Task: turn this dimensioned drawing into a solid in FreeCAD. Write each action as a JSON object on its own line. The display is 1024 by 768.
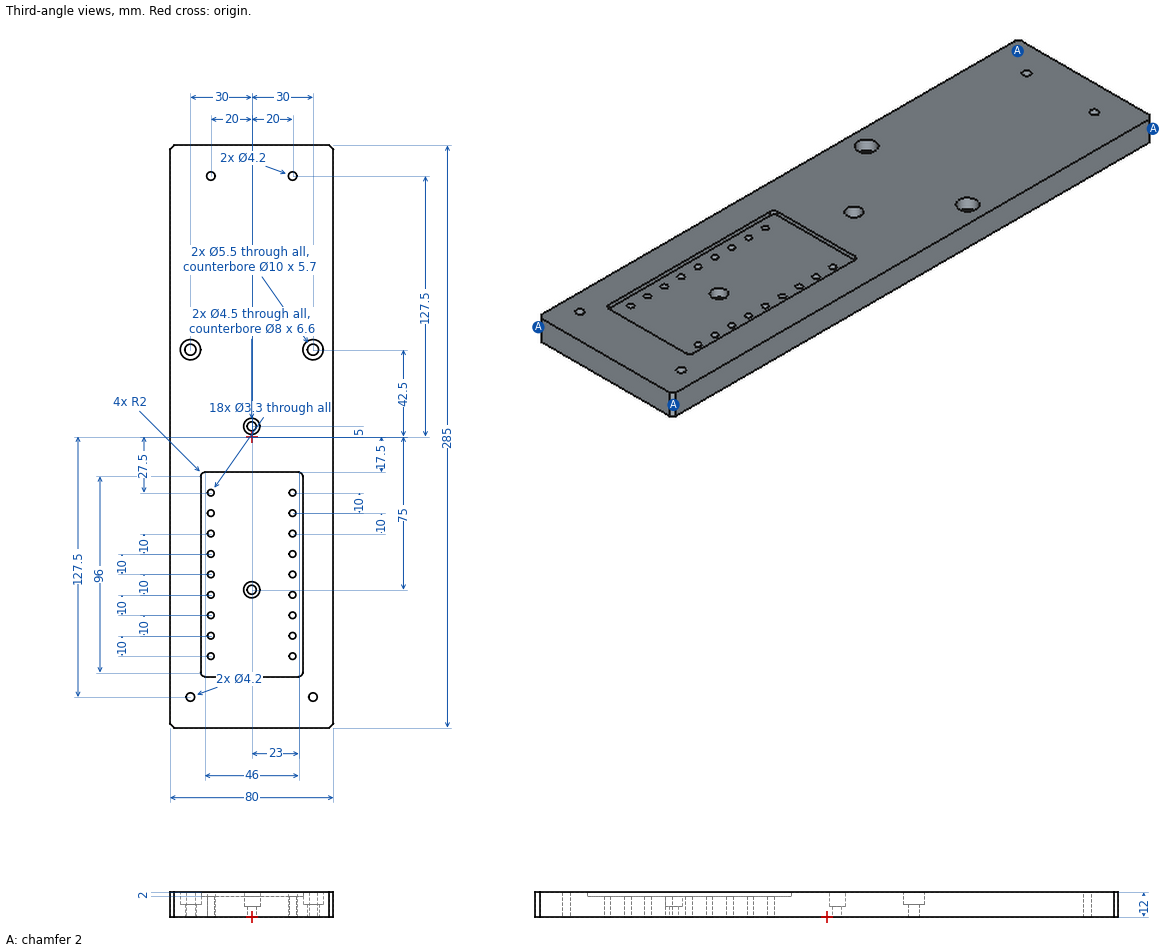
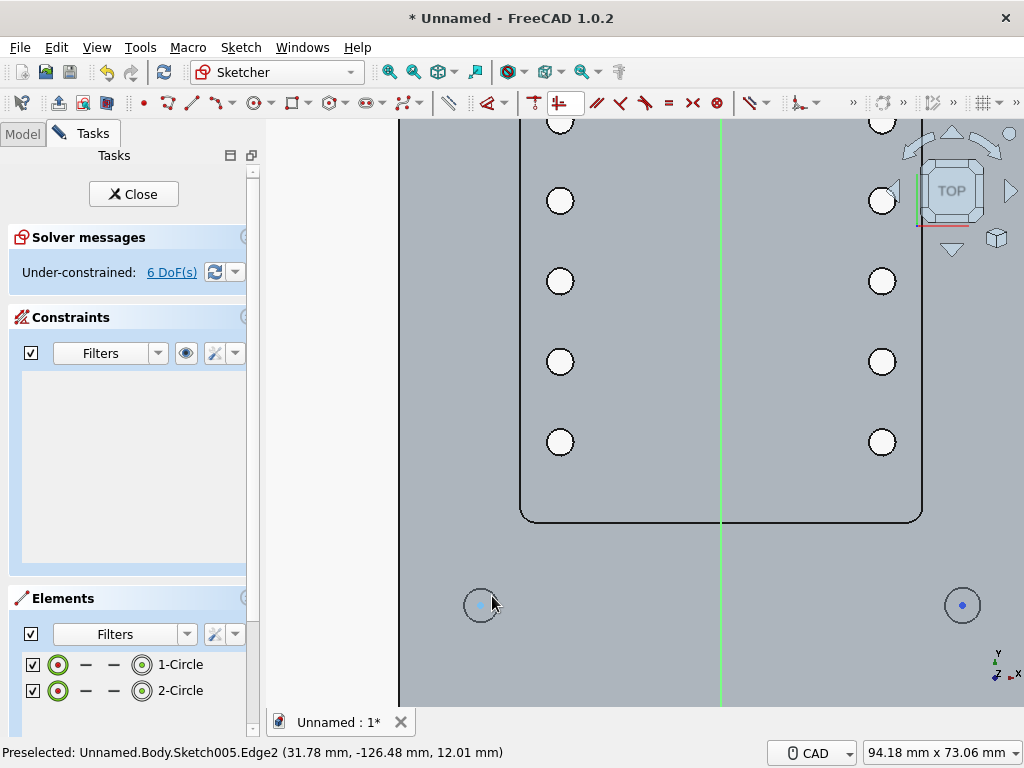
{"action": "left_click", "coordinate": [493, 594]}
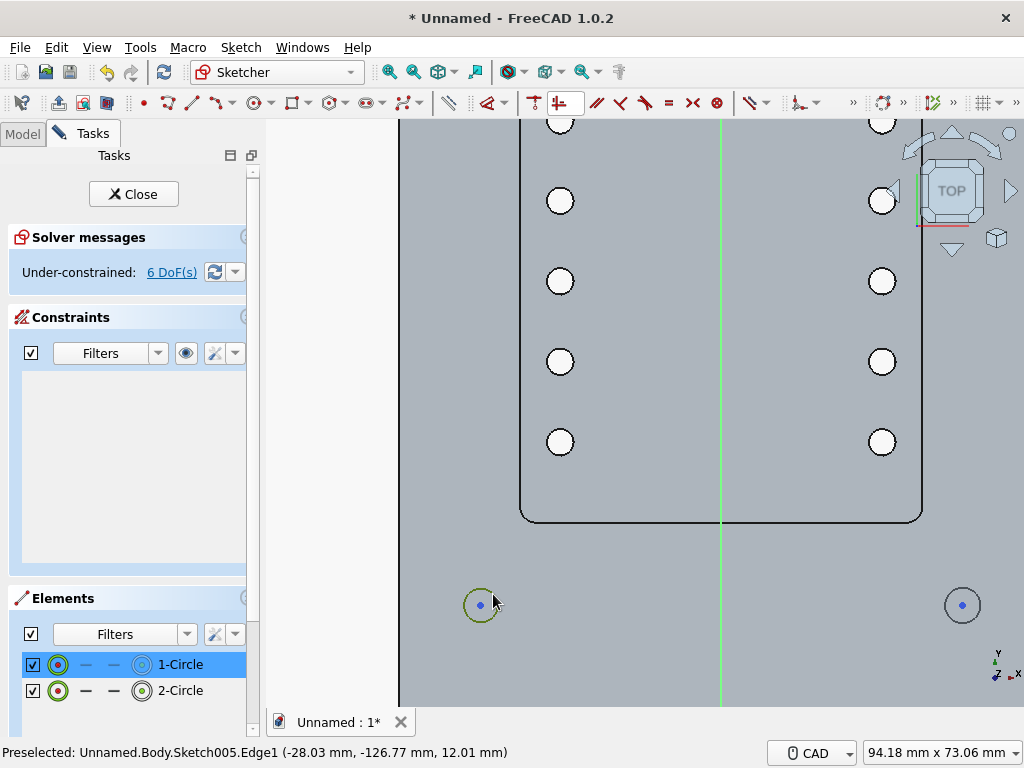
{"action": "scroll", "coordinate": [492, 596], "scroll_direction": "down", "scroll_amount": 5}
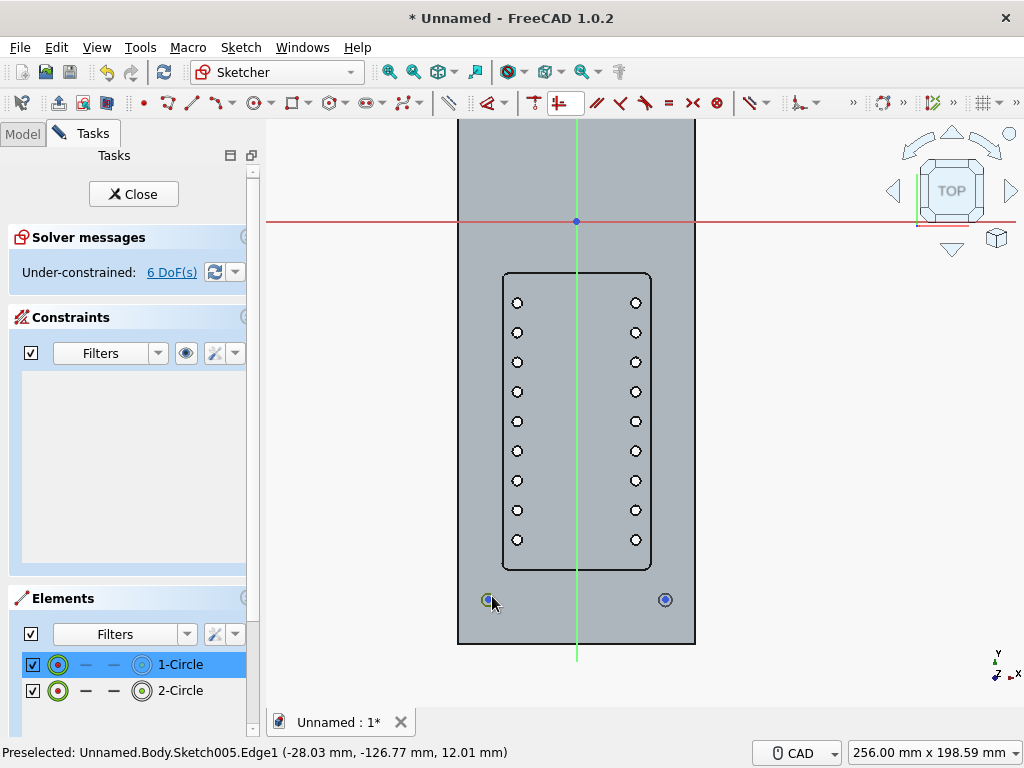
{"action": "scroll", "coordinate": [670, 595], "scroll_direction": "up", "scroll_amount": 4}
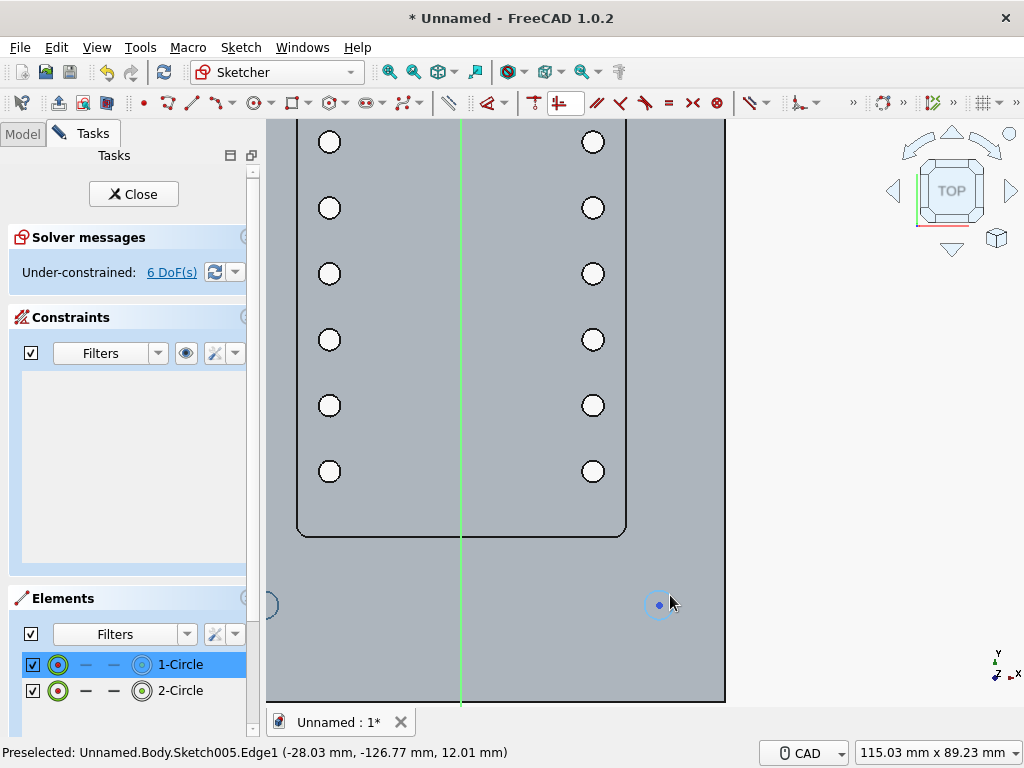
{"action": "left_click", "coordinate": [669, 595]}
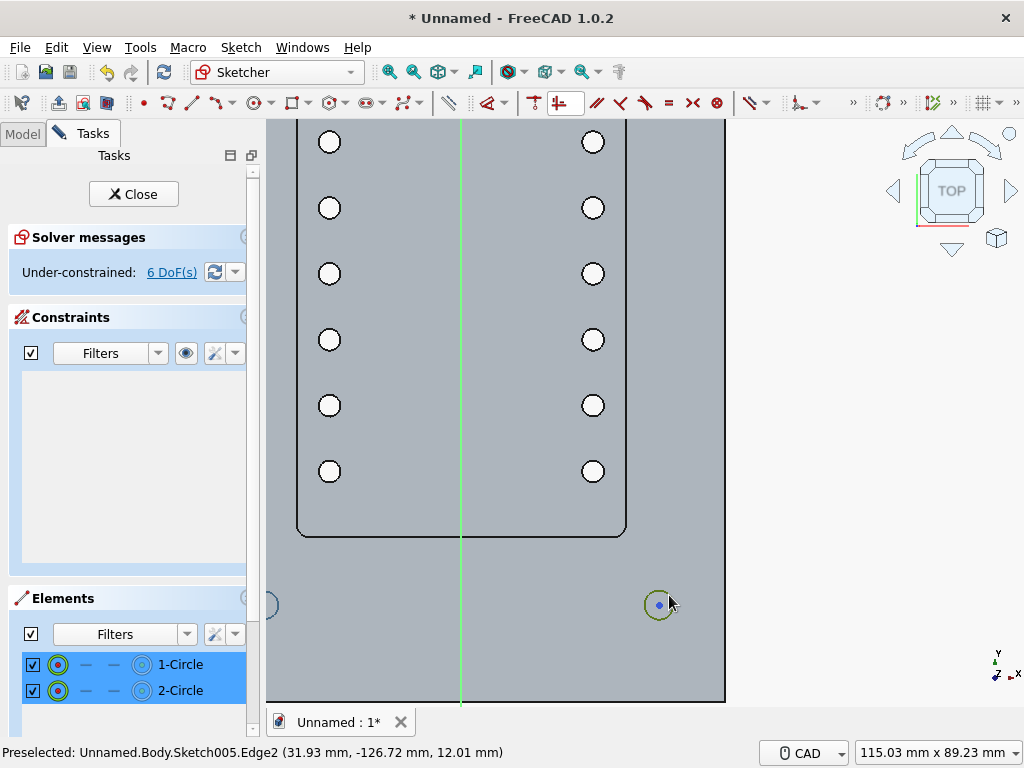
{"action": "key", "text": "e"}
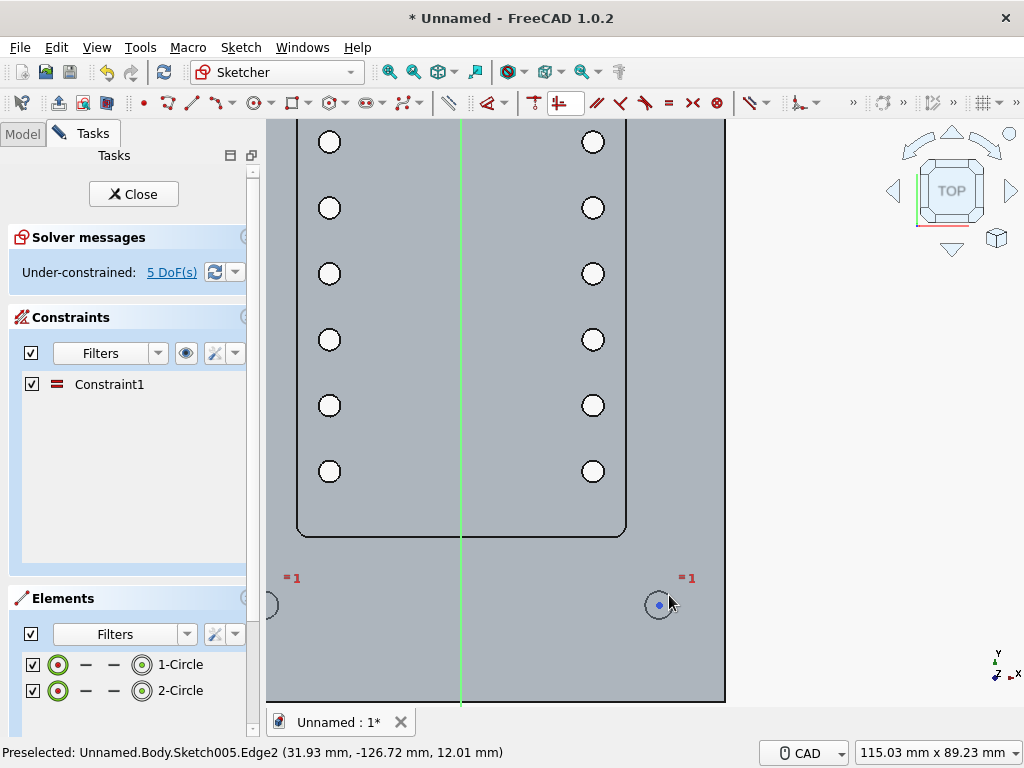
{"action": "scroll", "coordinate": [670, 595], "scroll_direction": "down", "scroll_amount": 4}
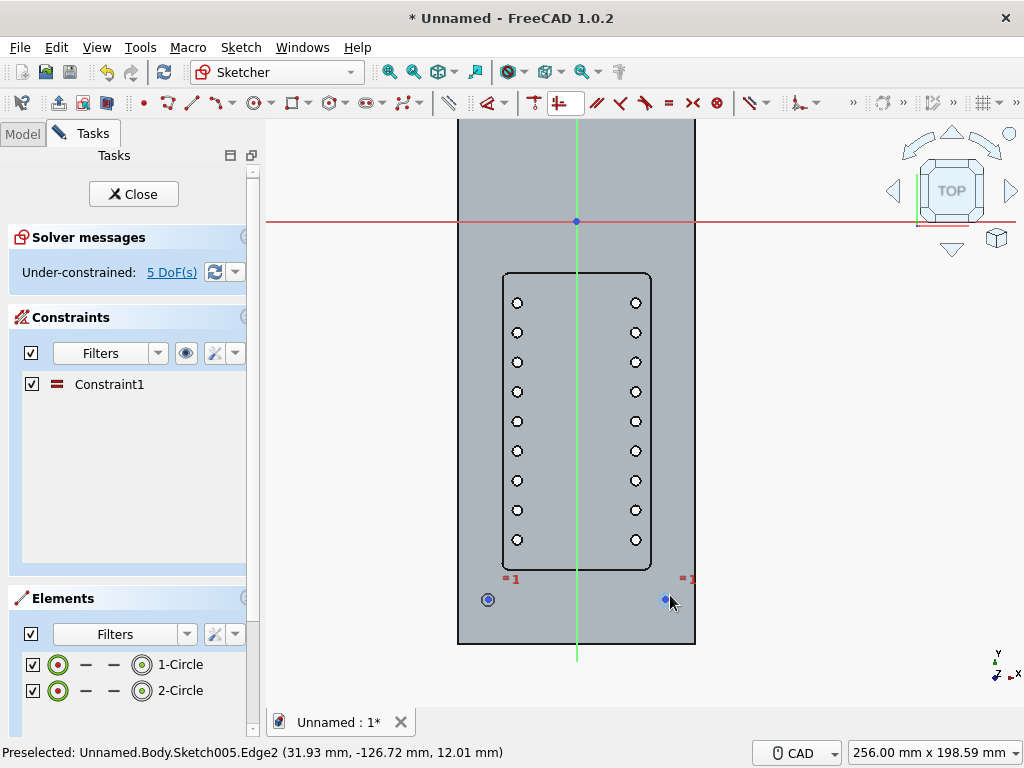
{"action": "left_click", "coordinate": [488, 600]}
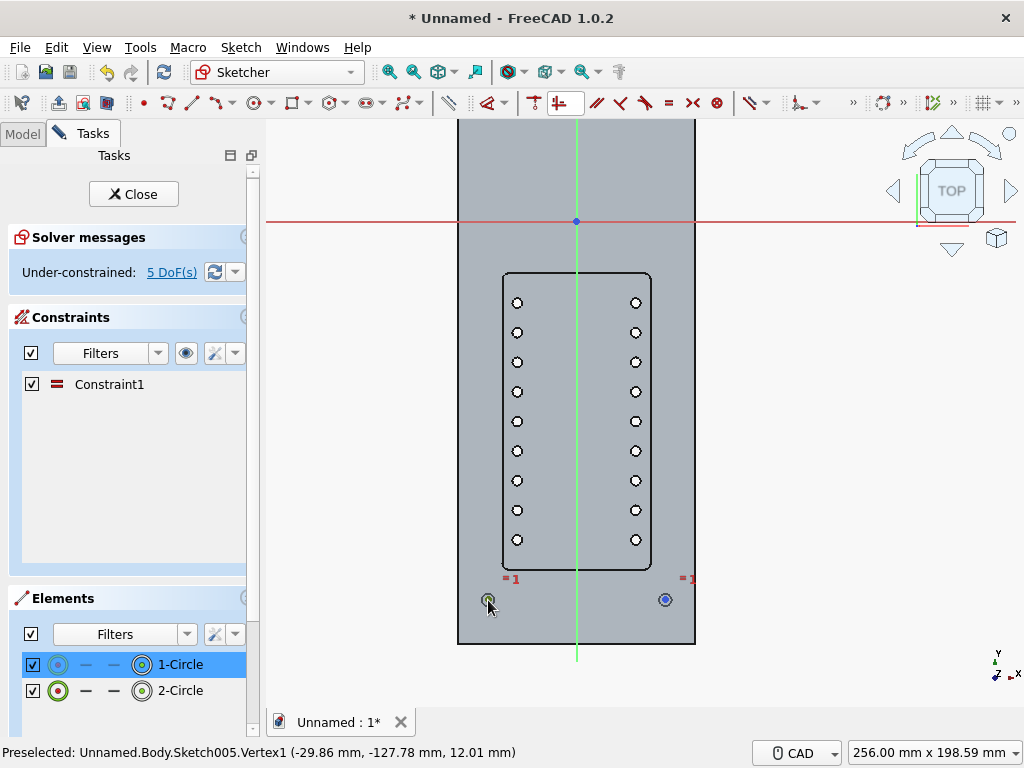
{"action": "left_click", "coordinate": [665, 600]}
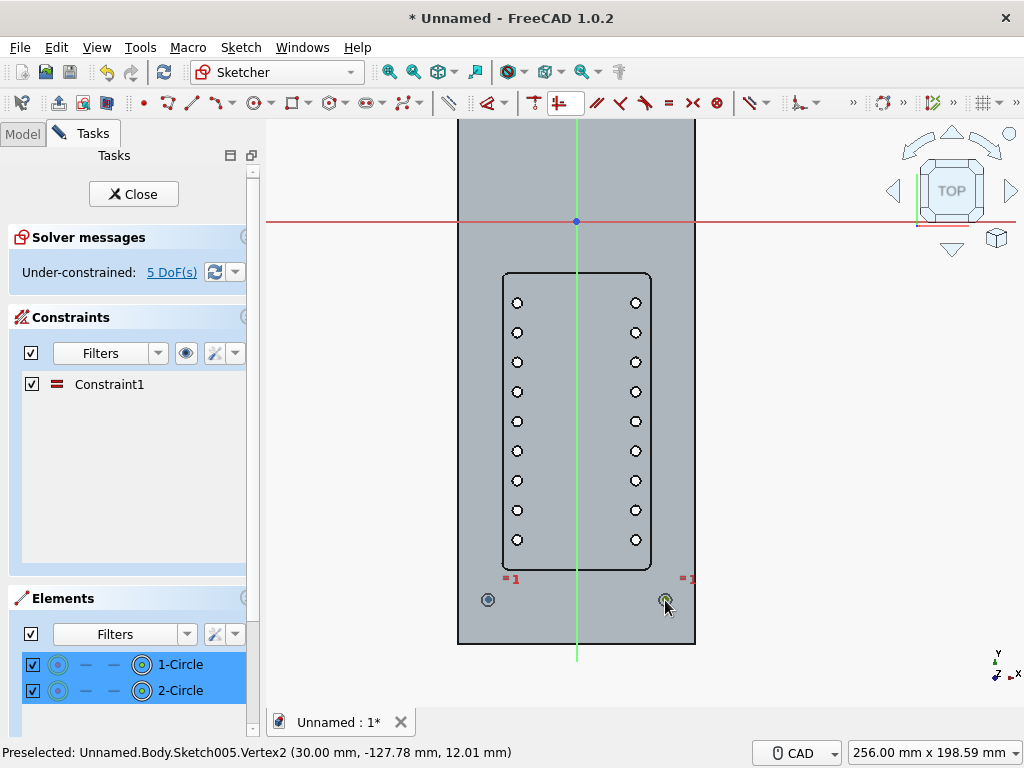
{"action": "key", "text": "h"}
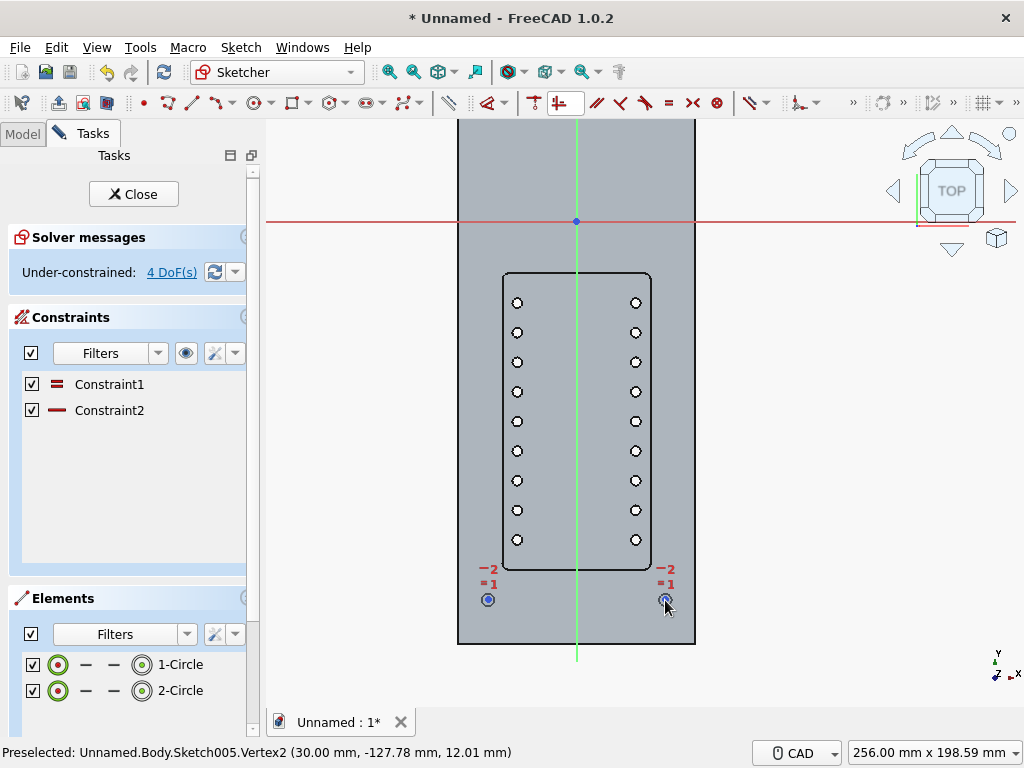
{"action": "key", "text": "d"}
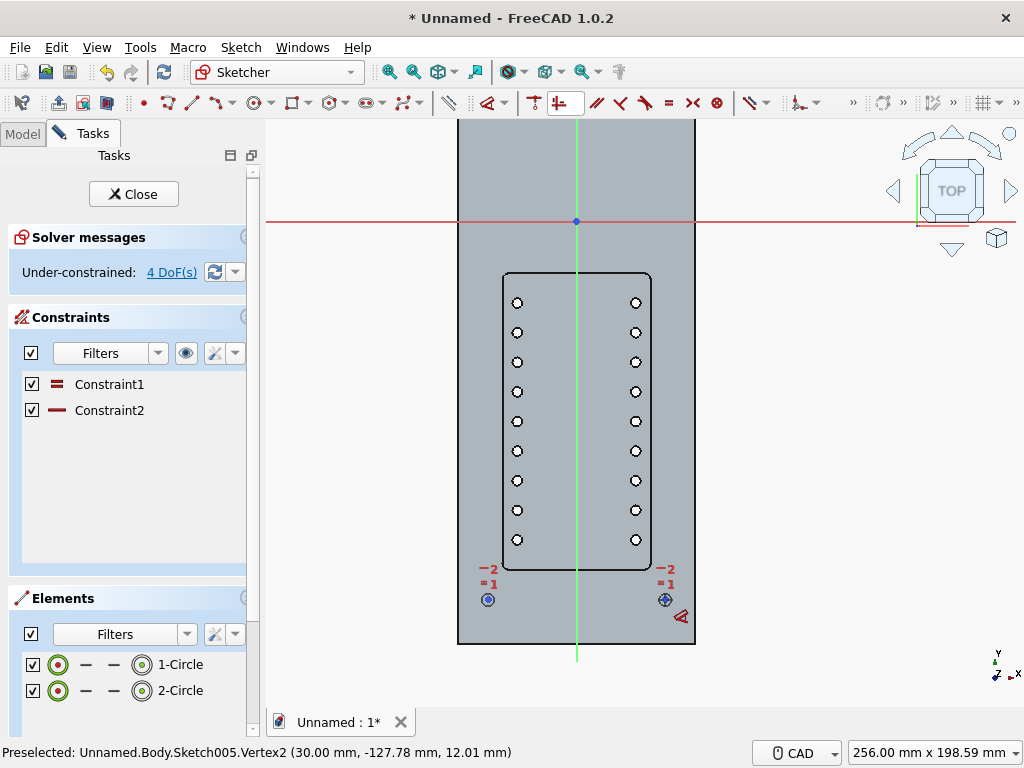
{"action": "scroll", "coordinate": [488, 606], "scroll_direction": "up", "scroll_amount": 6}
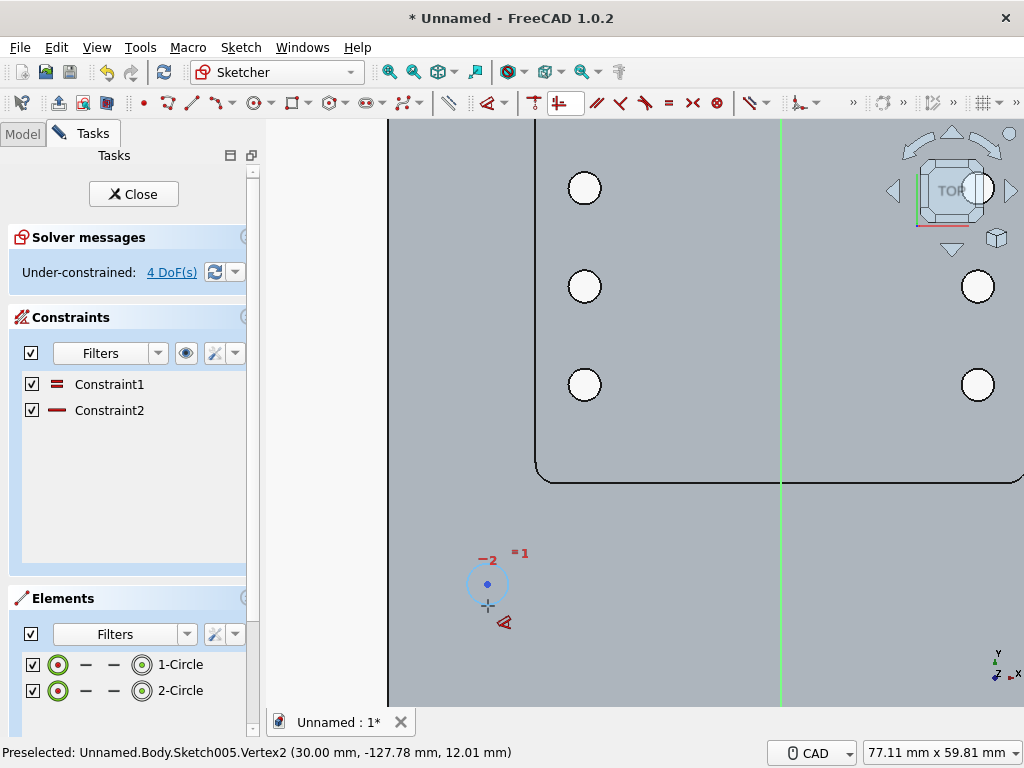
{"action": "left_click", "coordinate": [487, 605]}
{"action": "left_click", "coordinate": [486, 637]}